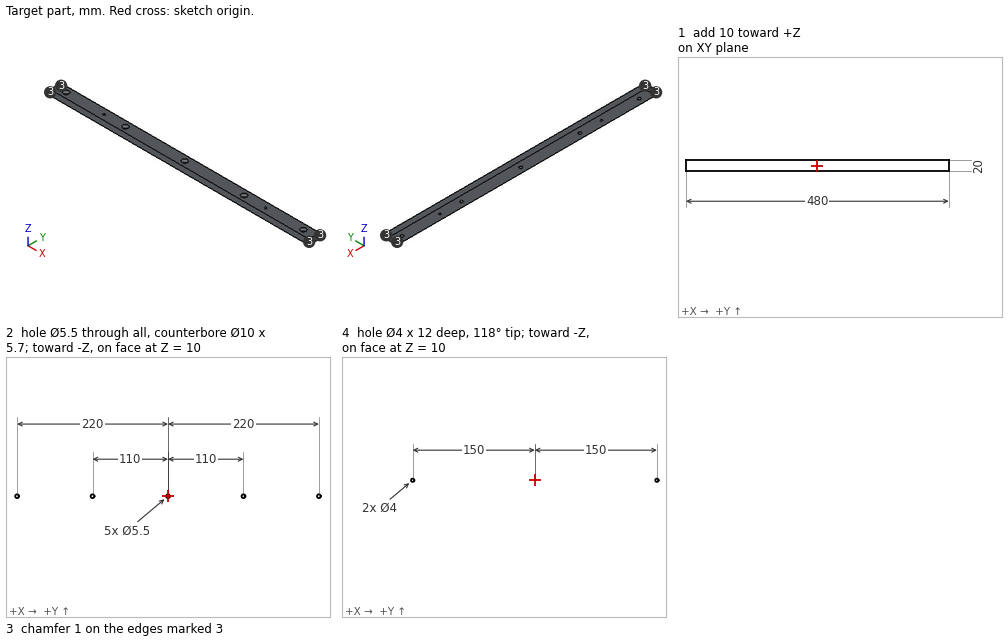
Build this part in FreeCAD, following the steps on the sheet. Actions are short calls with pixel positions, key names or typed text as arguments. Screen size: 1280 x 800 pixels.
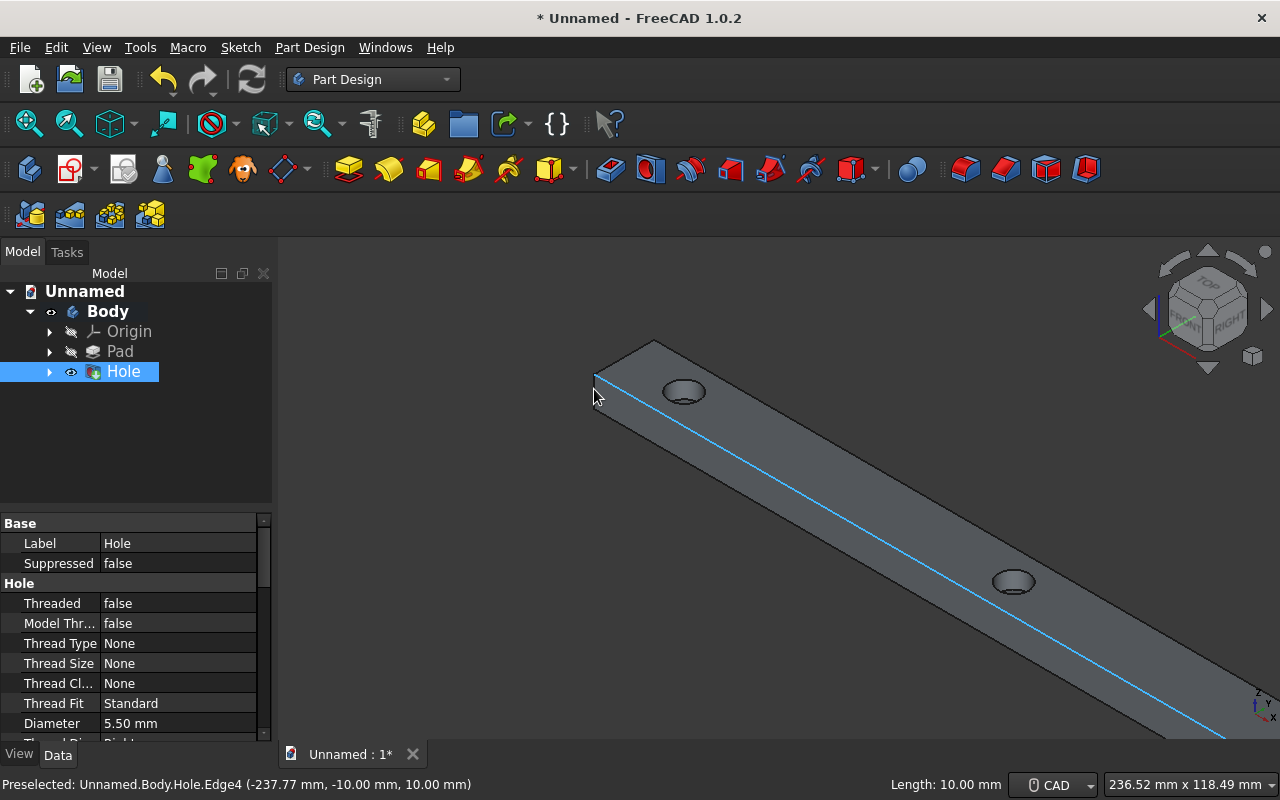
click(30, 124)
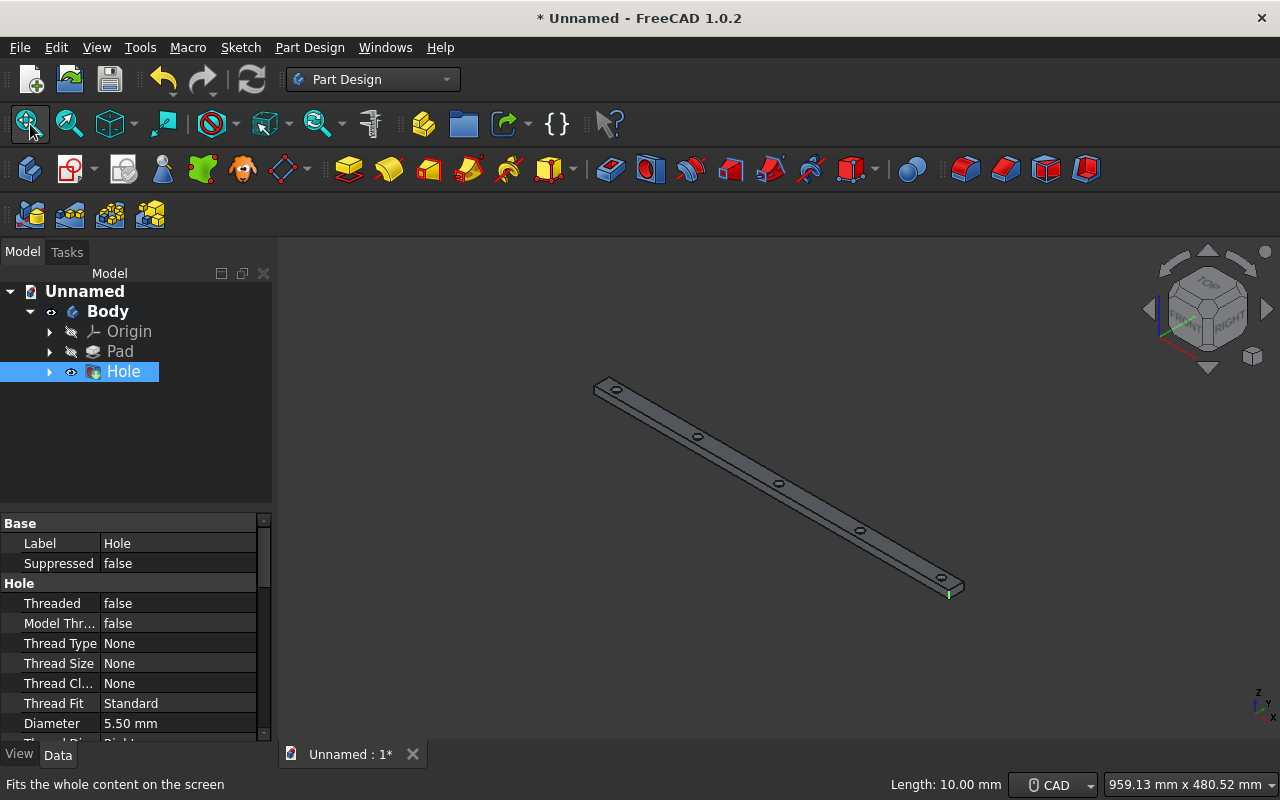
key(2)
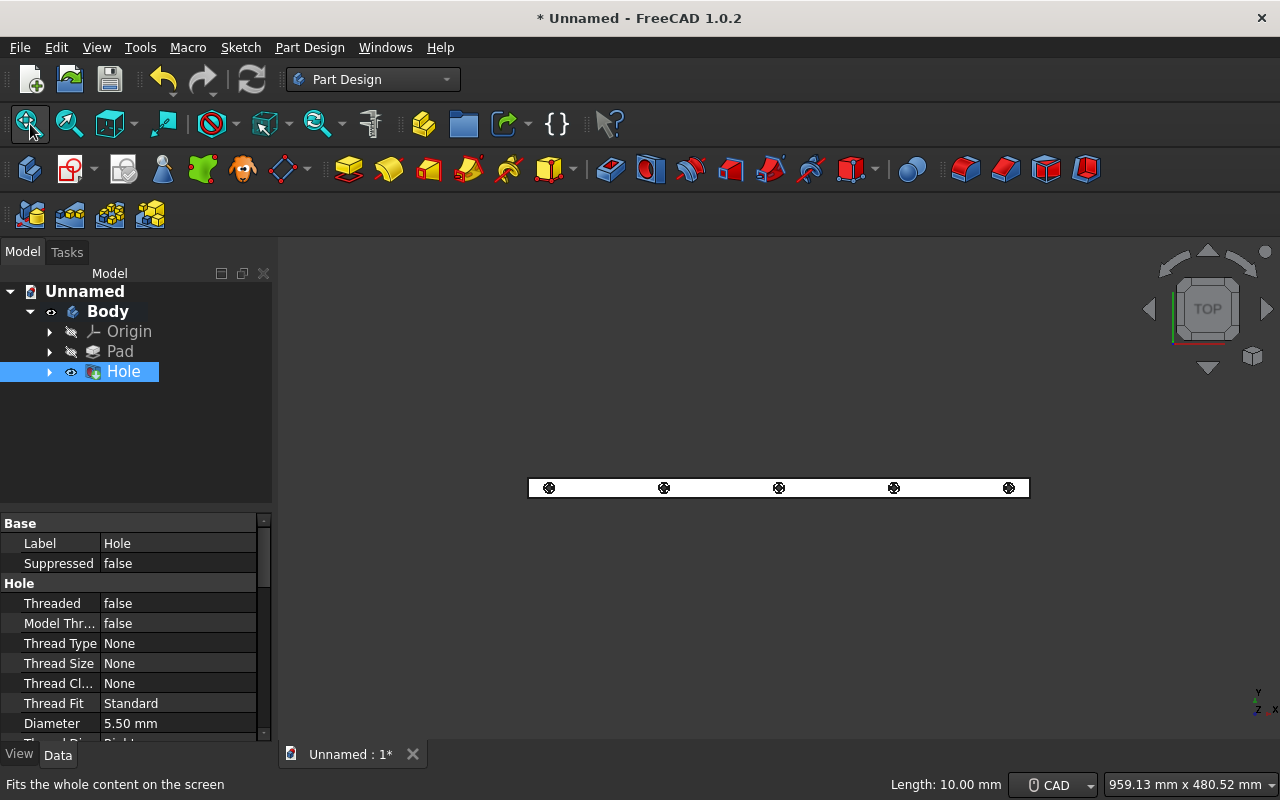
scroll(528, 497, up, 7)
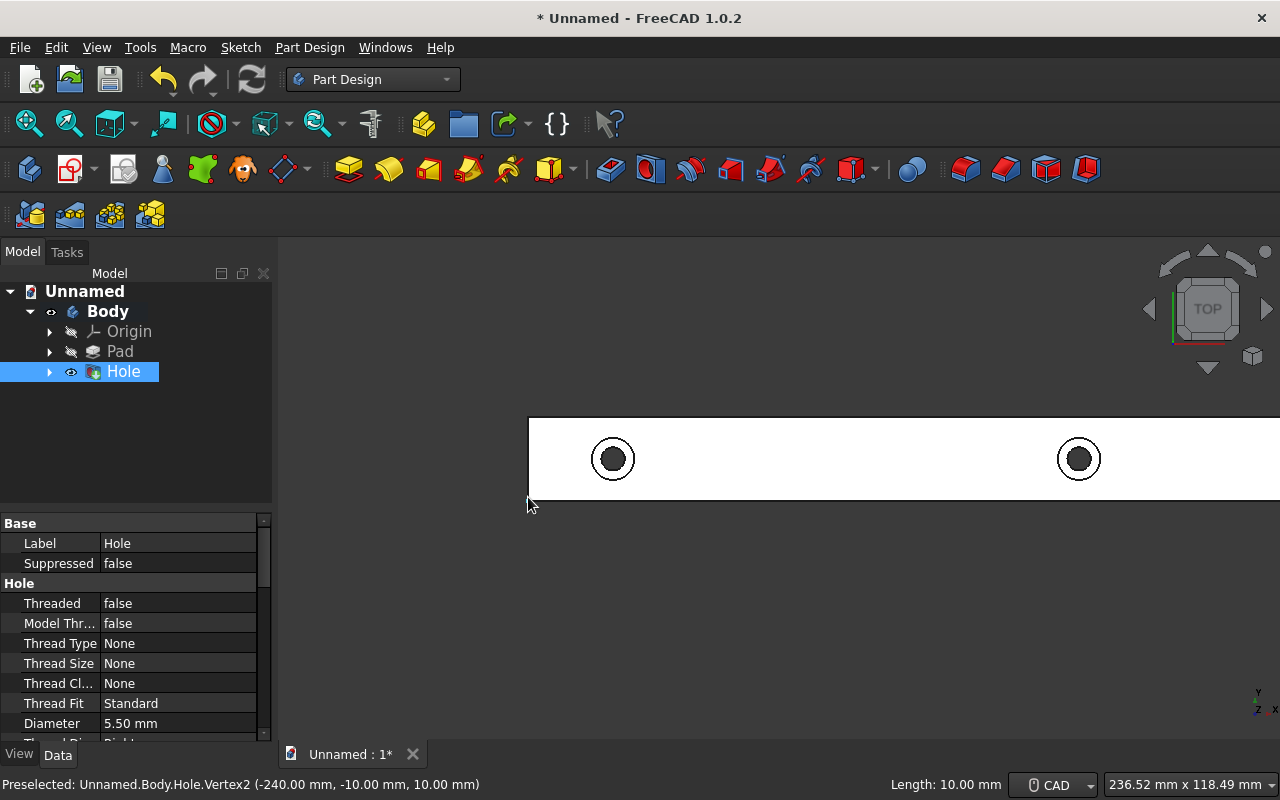
click(30, 124)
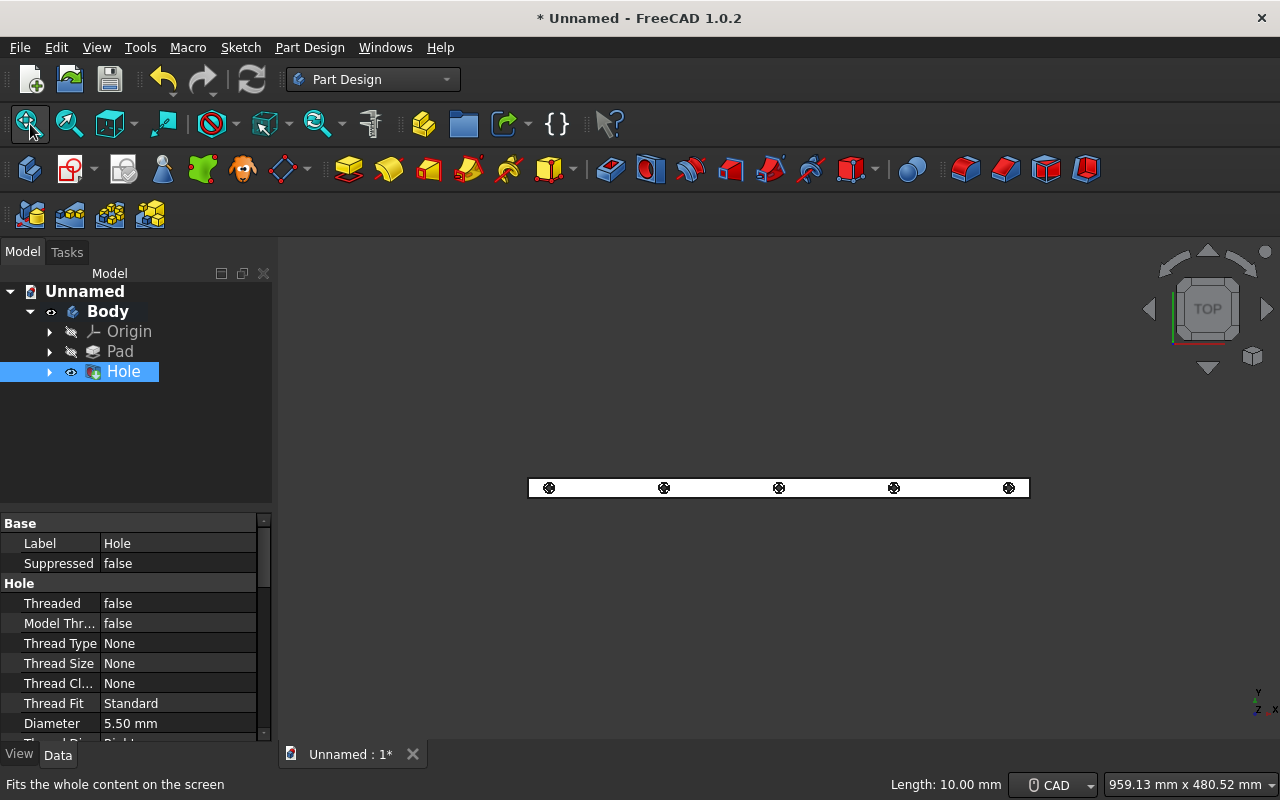
key(1)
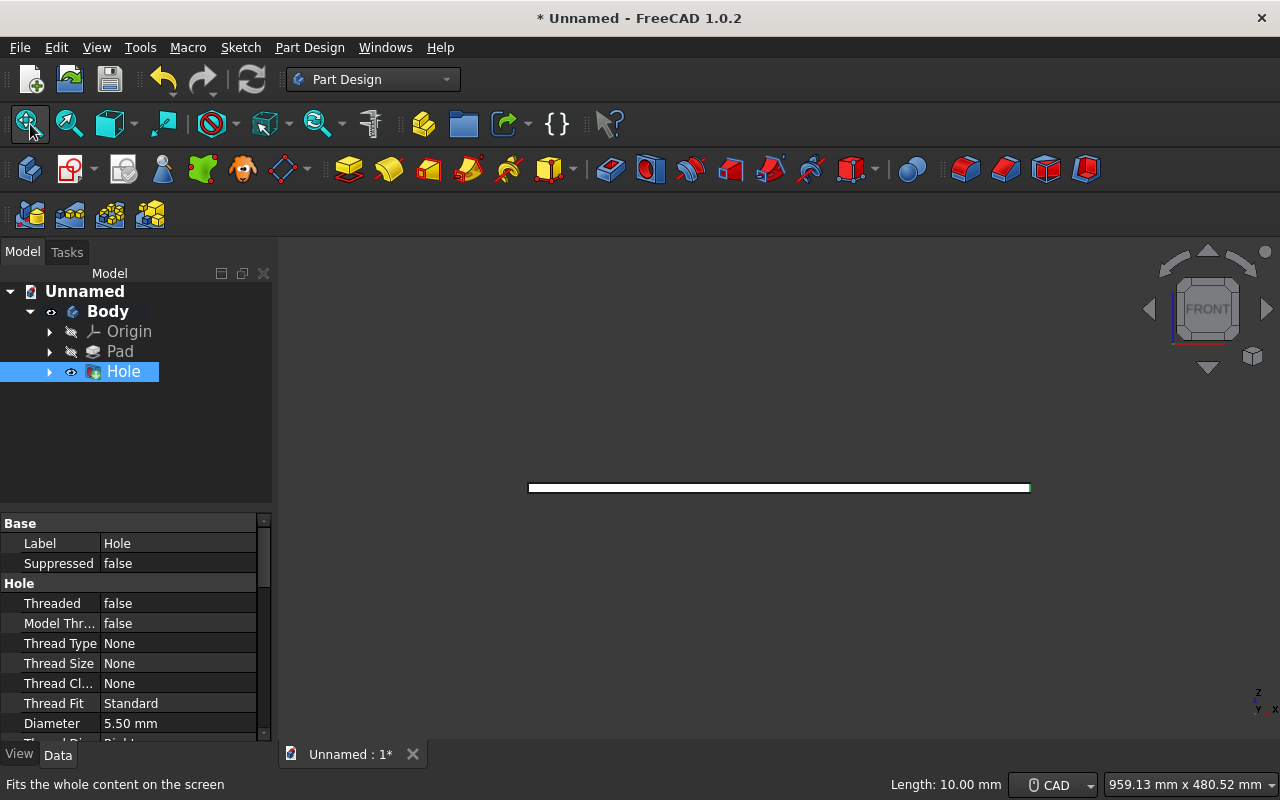
scroll(528, 487, up, 7)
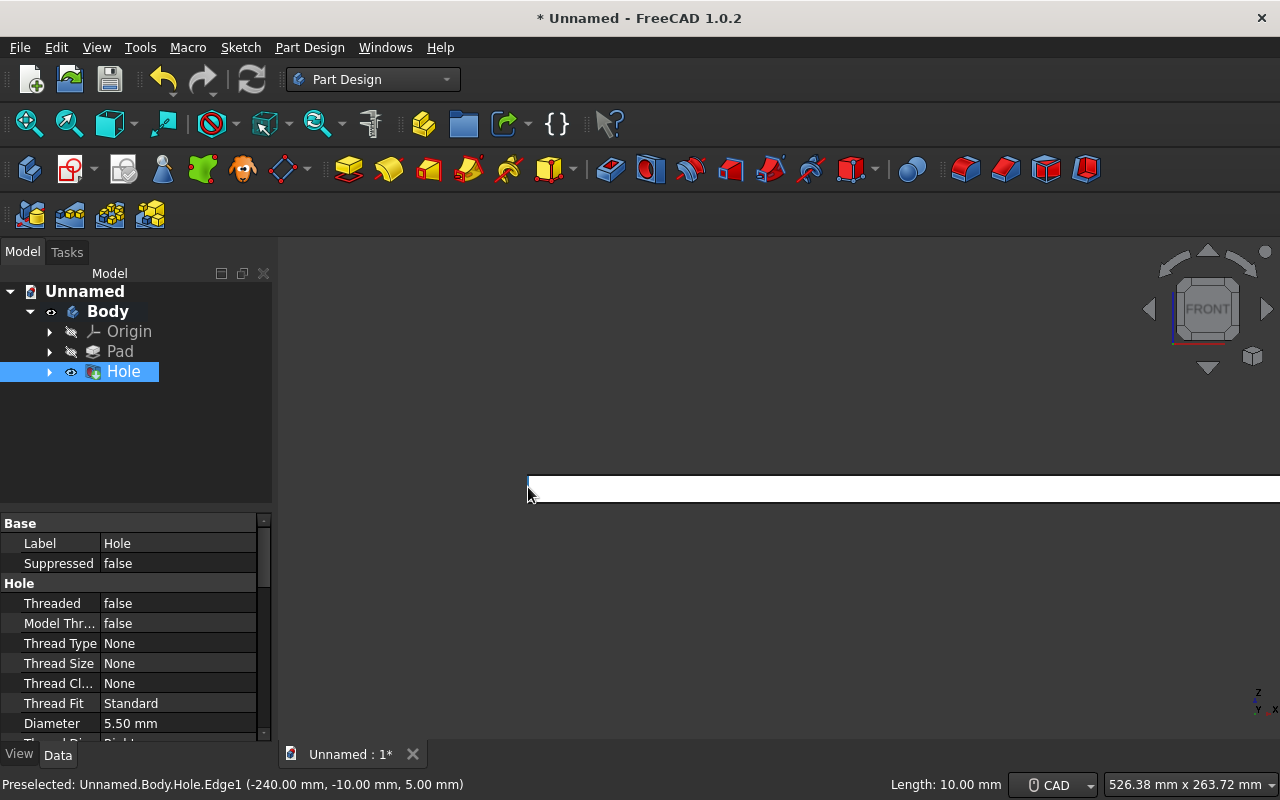
click(528, 489, ctrl)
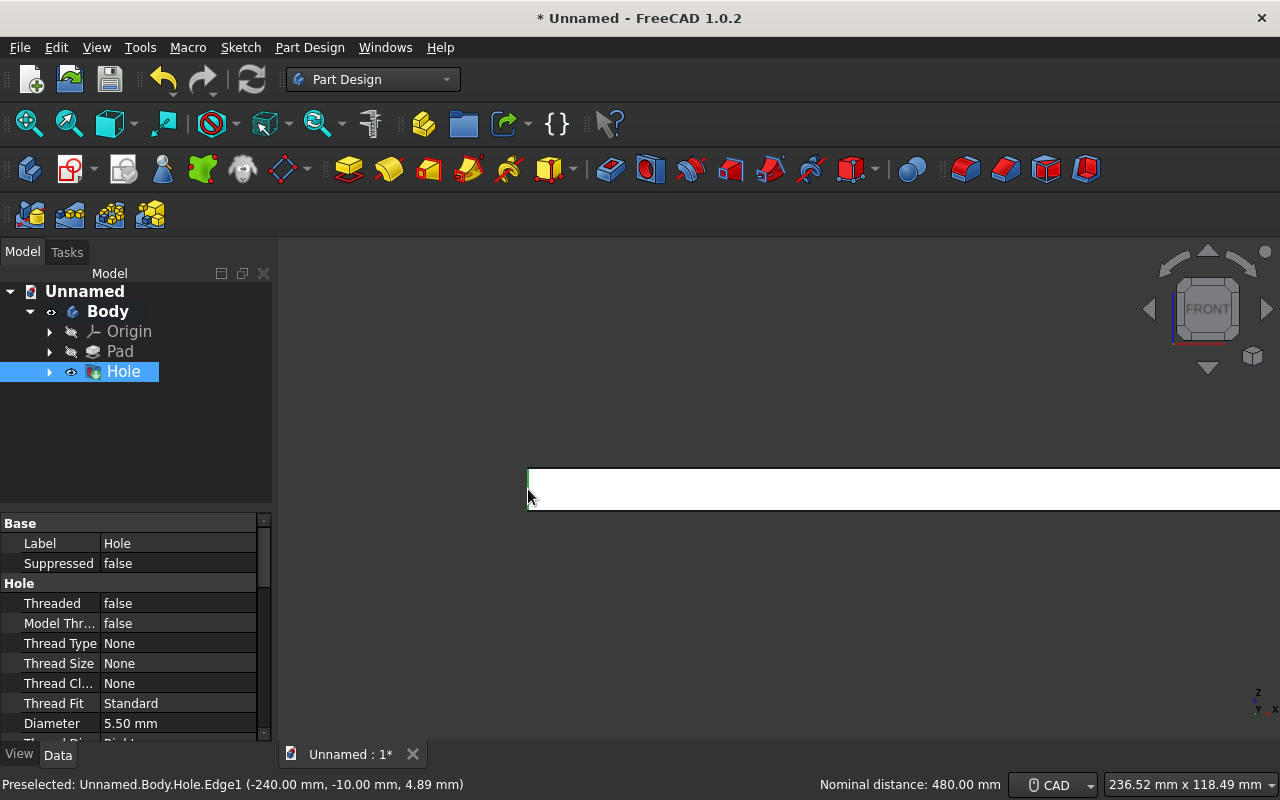
click(30, 124)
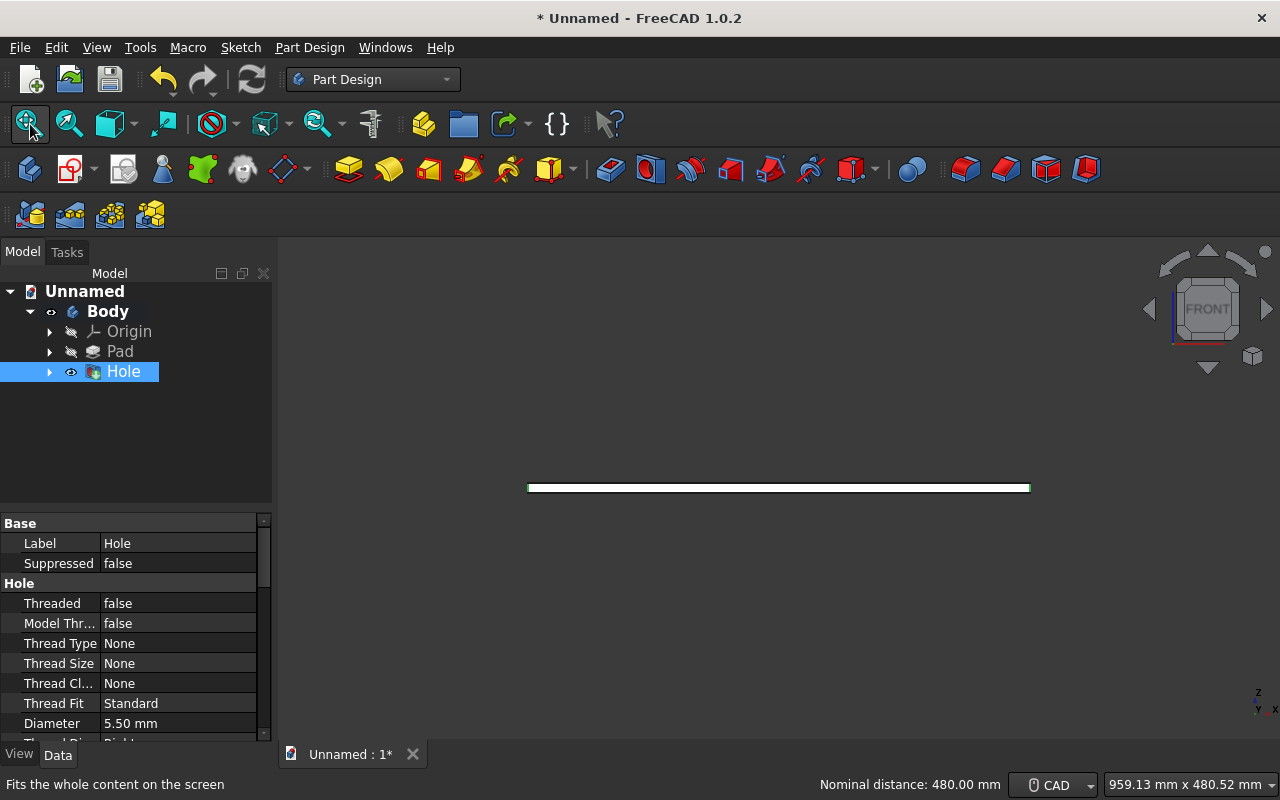
key(3)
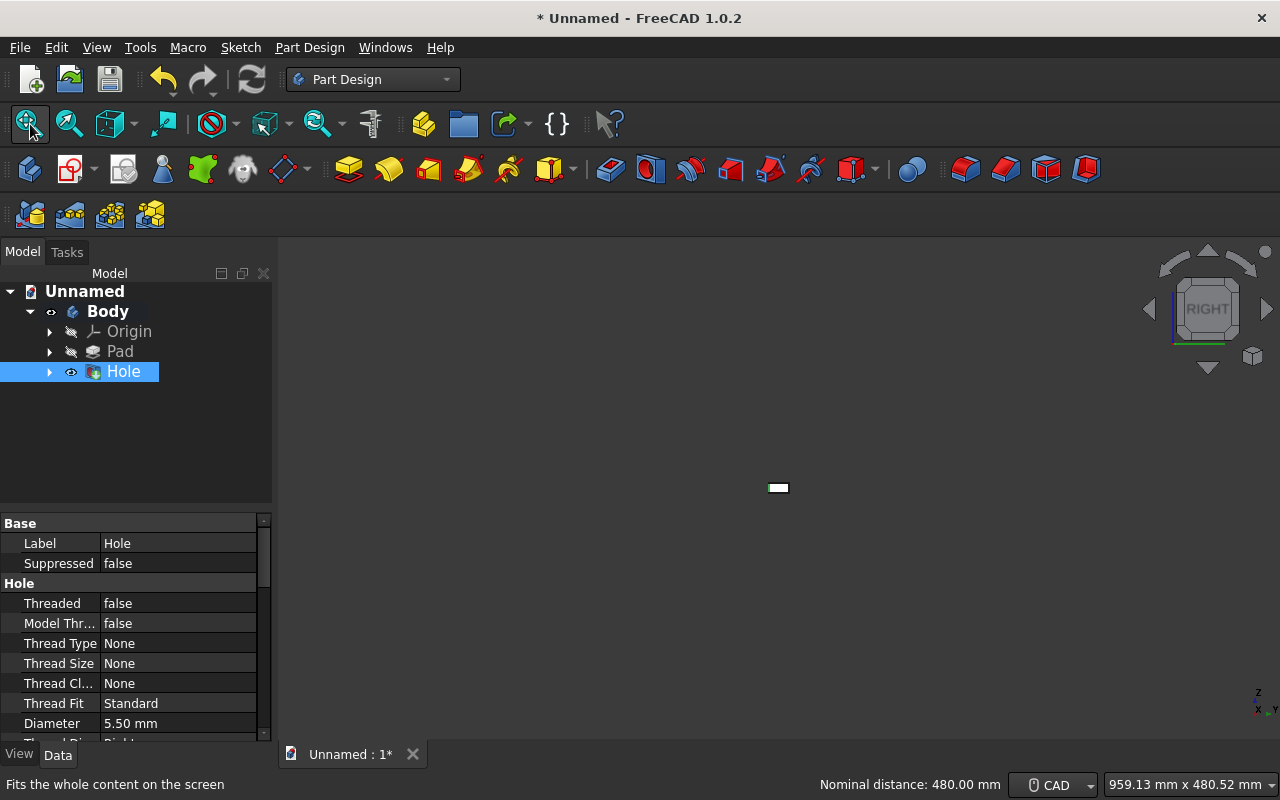
click(30, 124)